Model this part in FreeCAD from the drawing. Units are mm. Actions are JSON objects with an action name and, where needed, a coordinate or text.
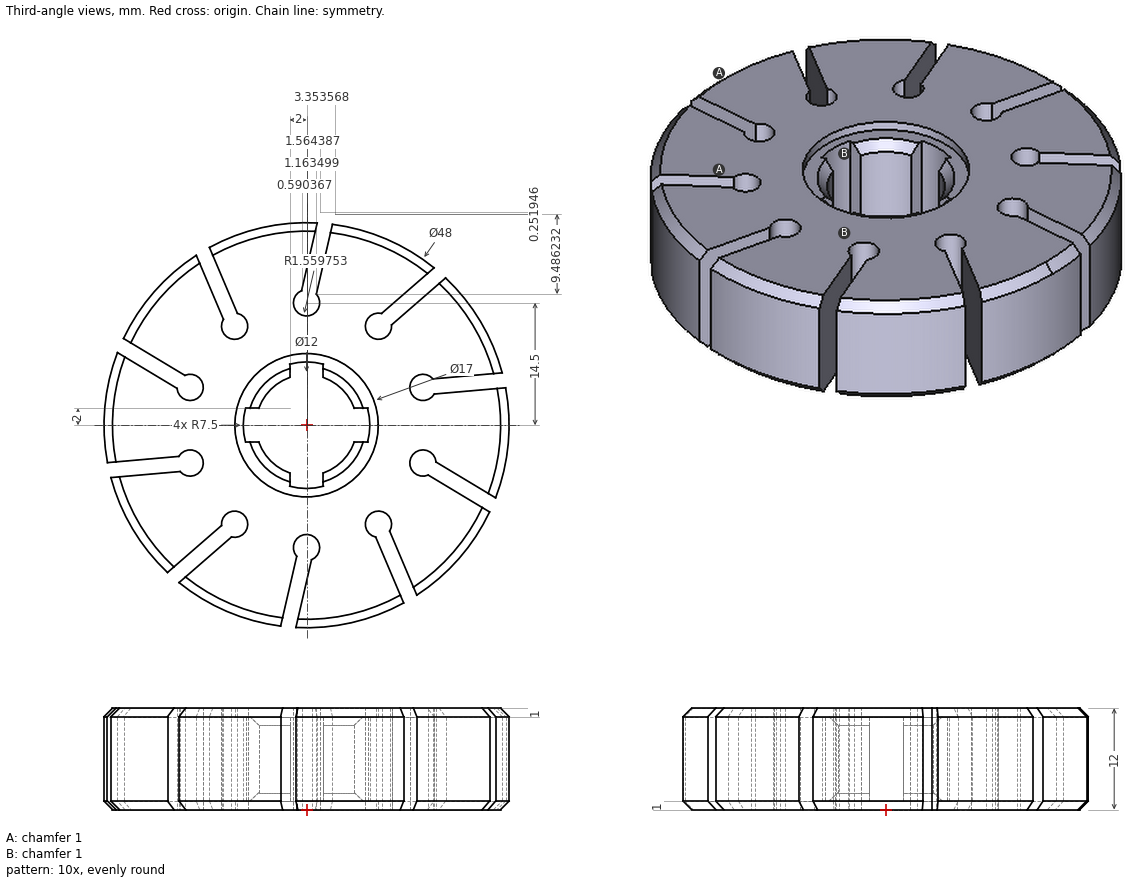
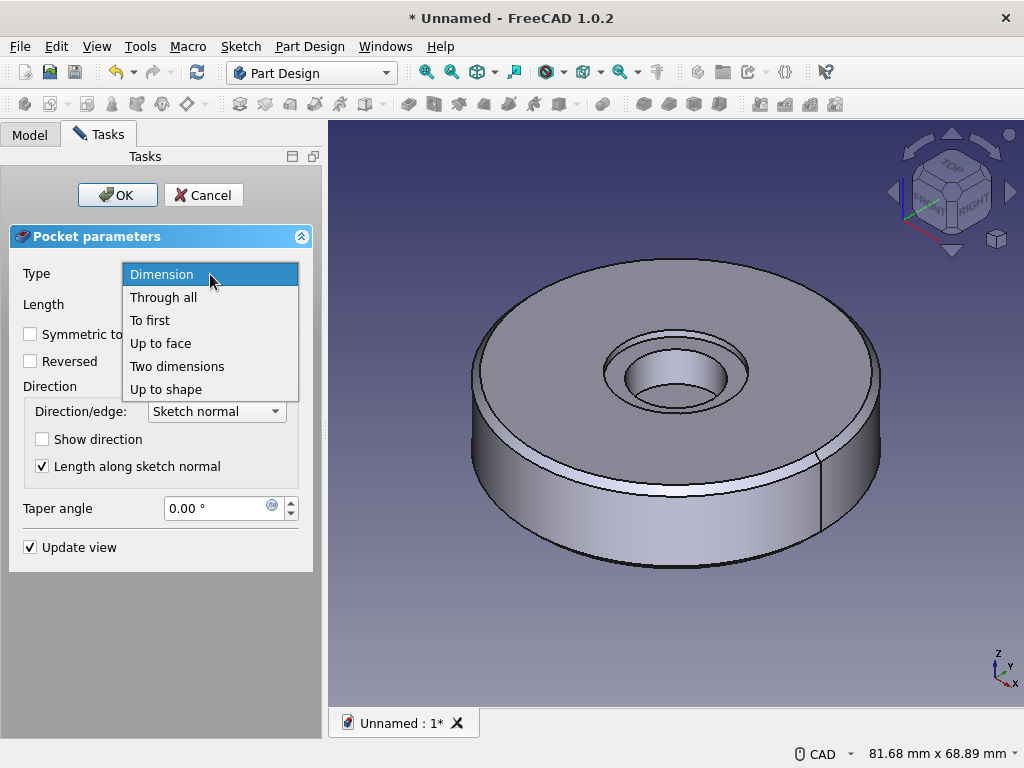
{"action": "left_click", "coordinate": [208, 298]}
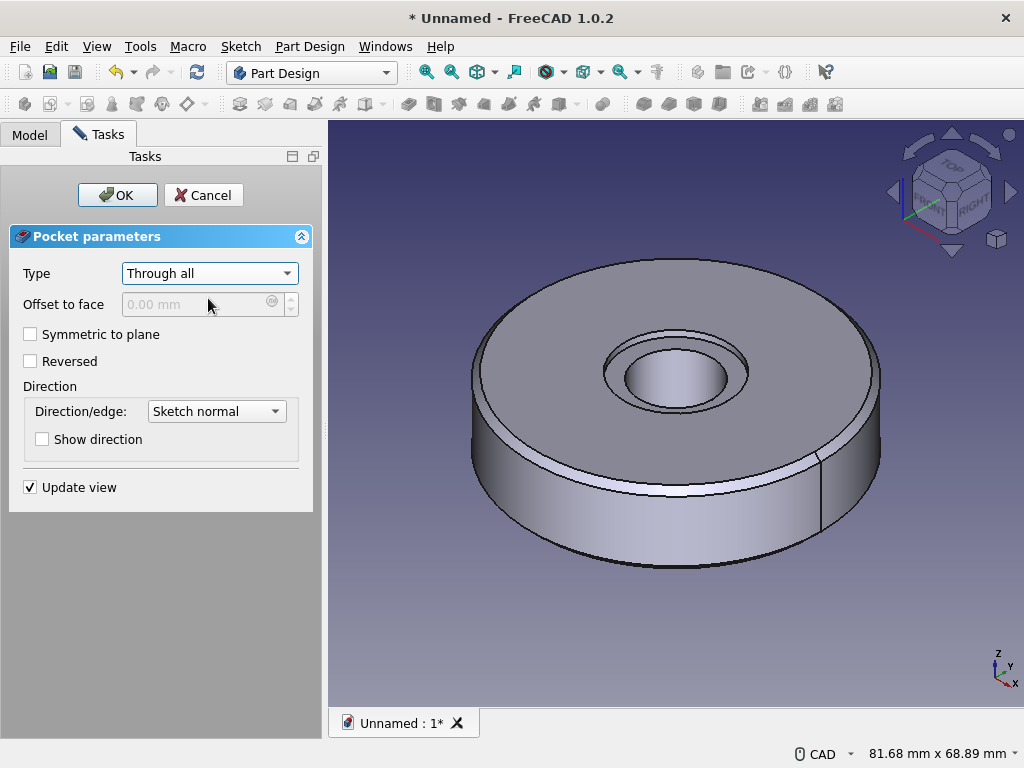
{"action": "left_click", "coordinate": [118, 195]}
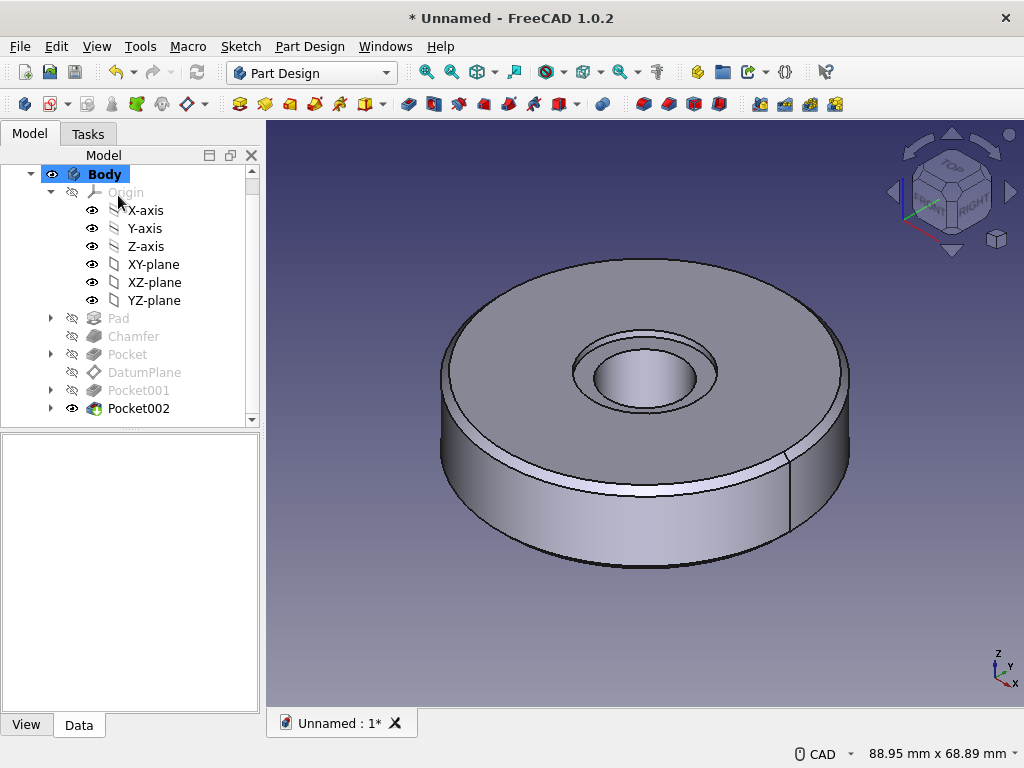
{"action": "left_click", "coordinate": [609, 357]}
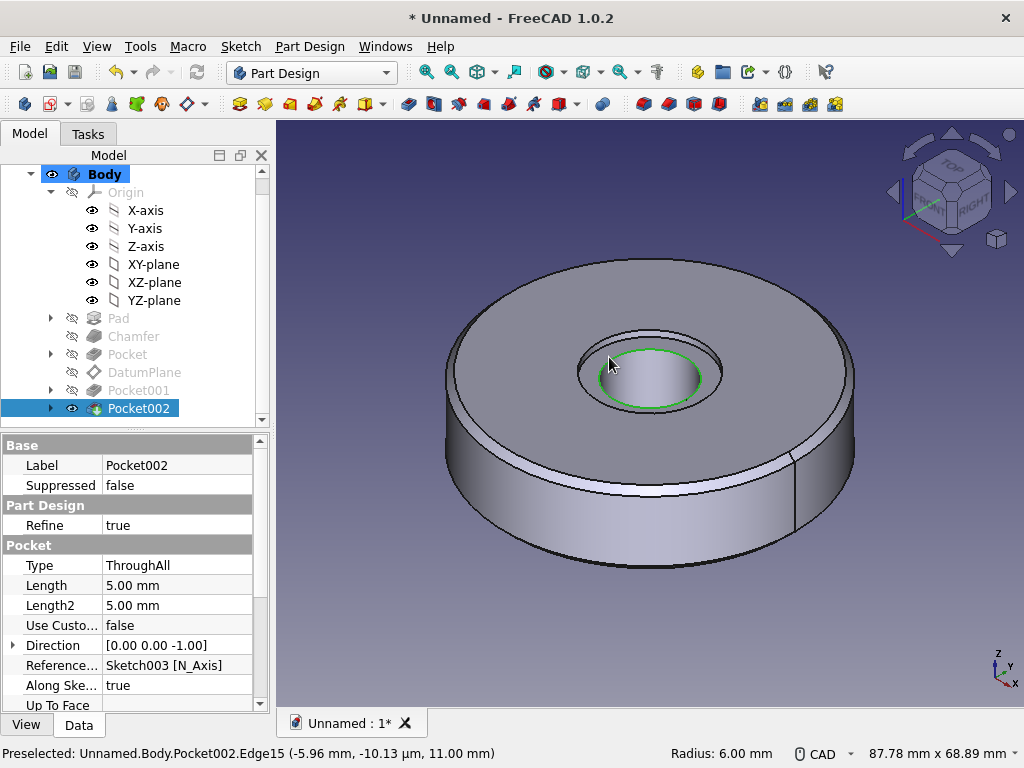
{"action": "key", "text": "2"}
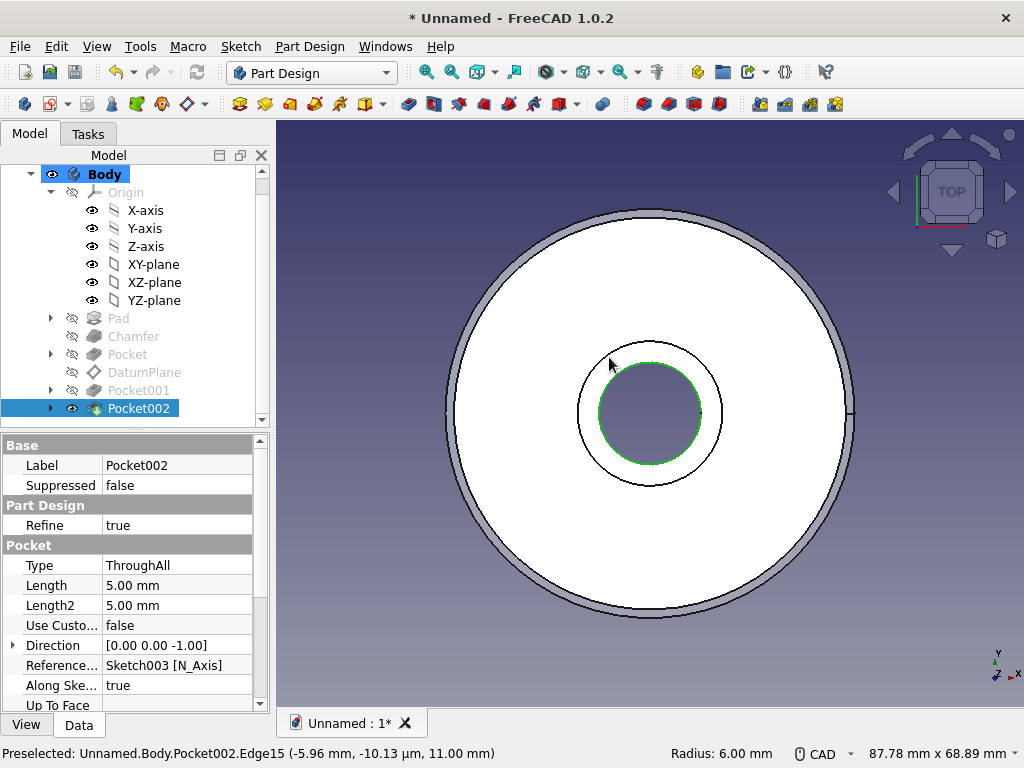
{"action": "key", "text": "0"}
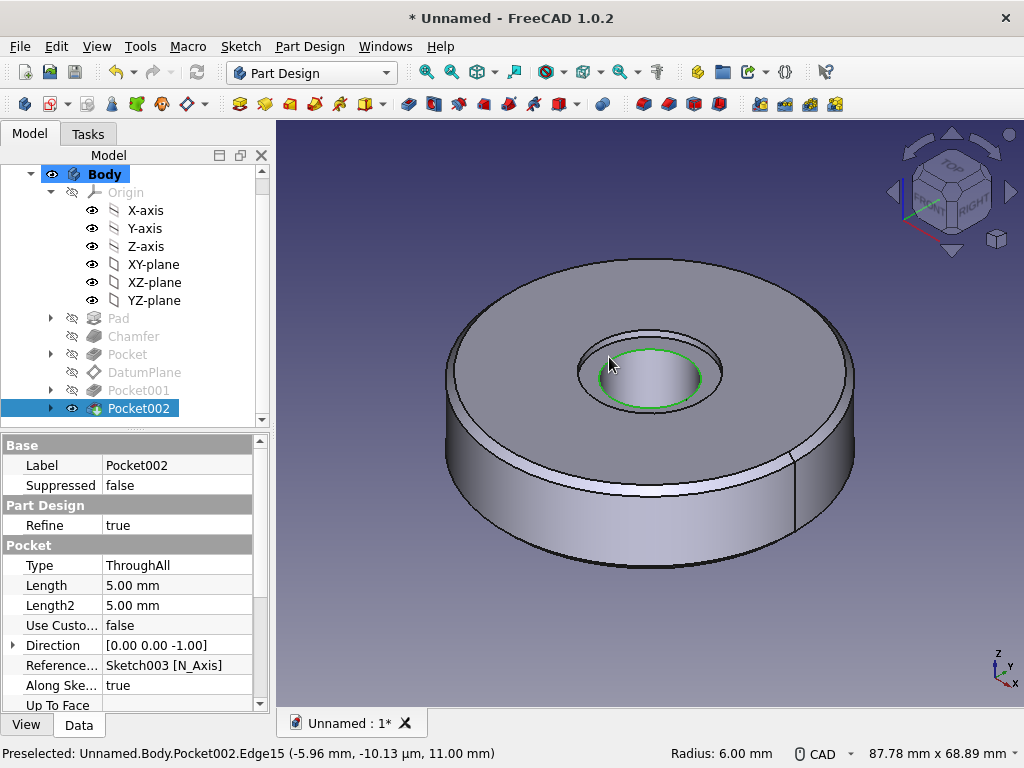
{"action": "key", "text": "1"}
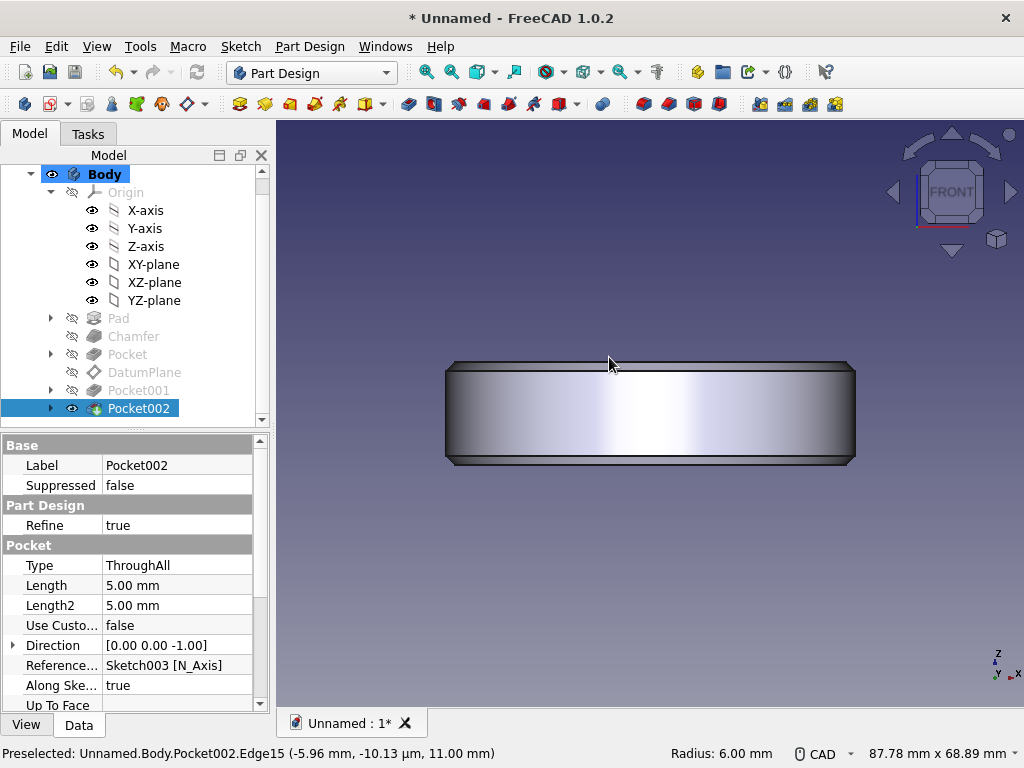
{"action": "key", "text": "3"}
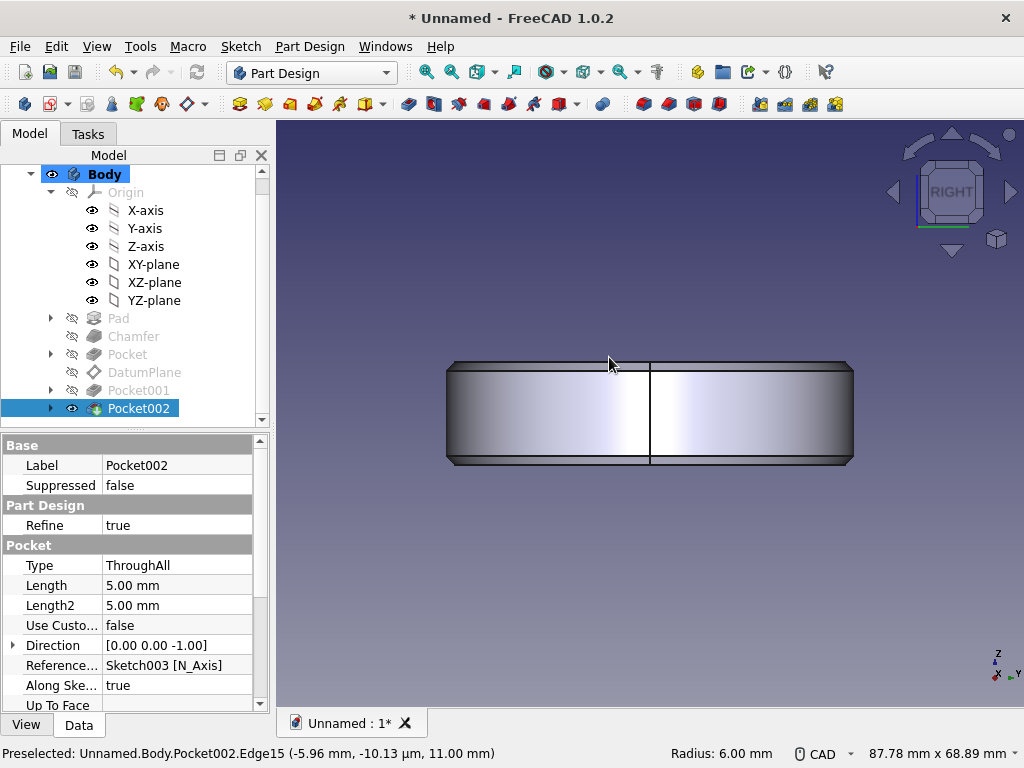
{"action": "key", "text": "5"}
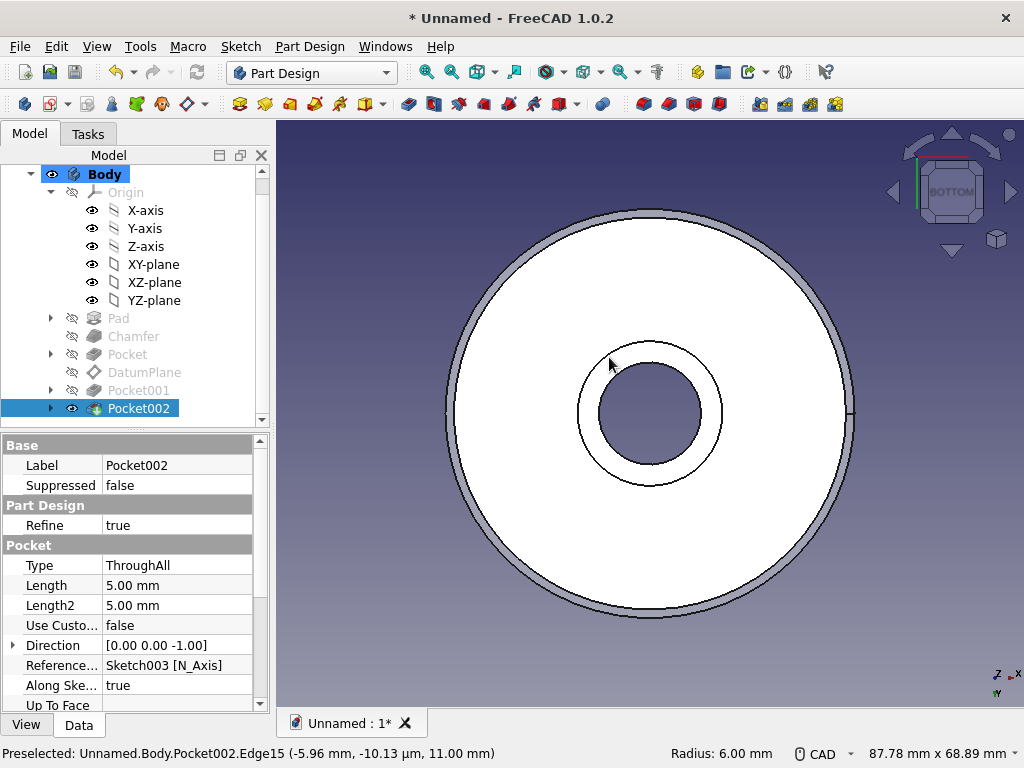
{"action": "left_click", "coordinate": [599, 413], "text": "ctrl"}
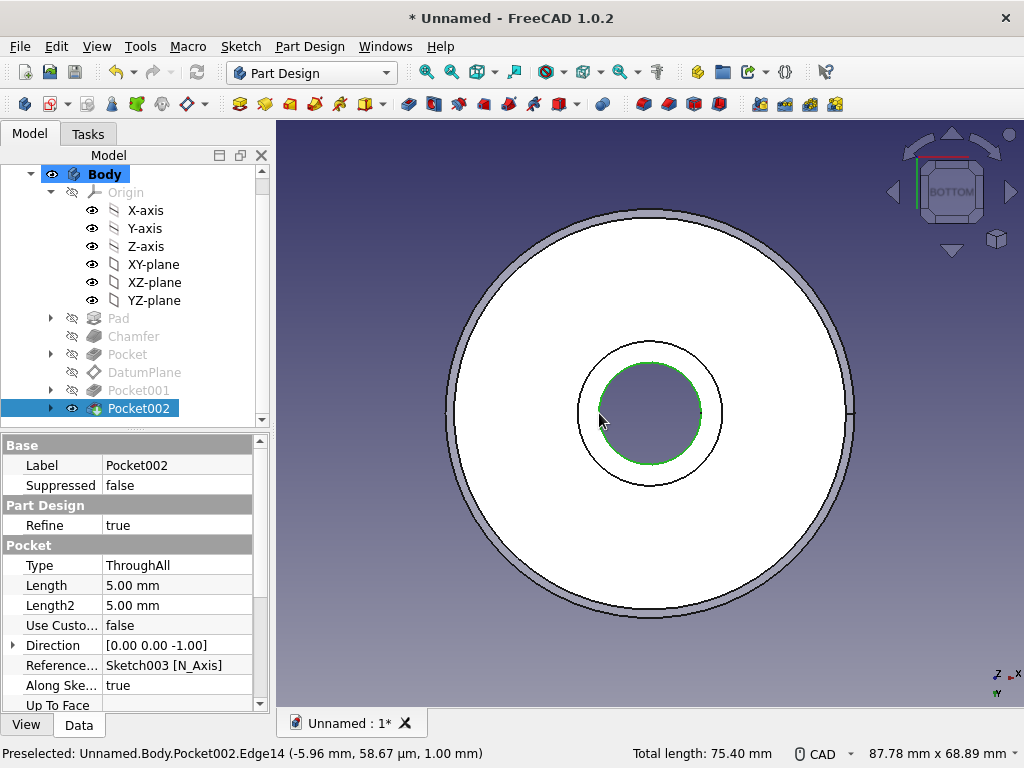
{"action": "left_click", "coordinate": [669, 104]}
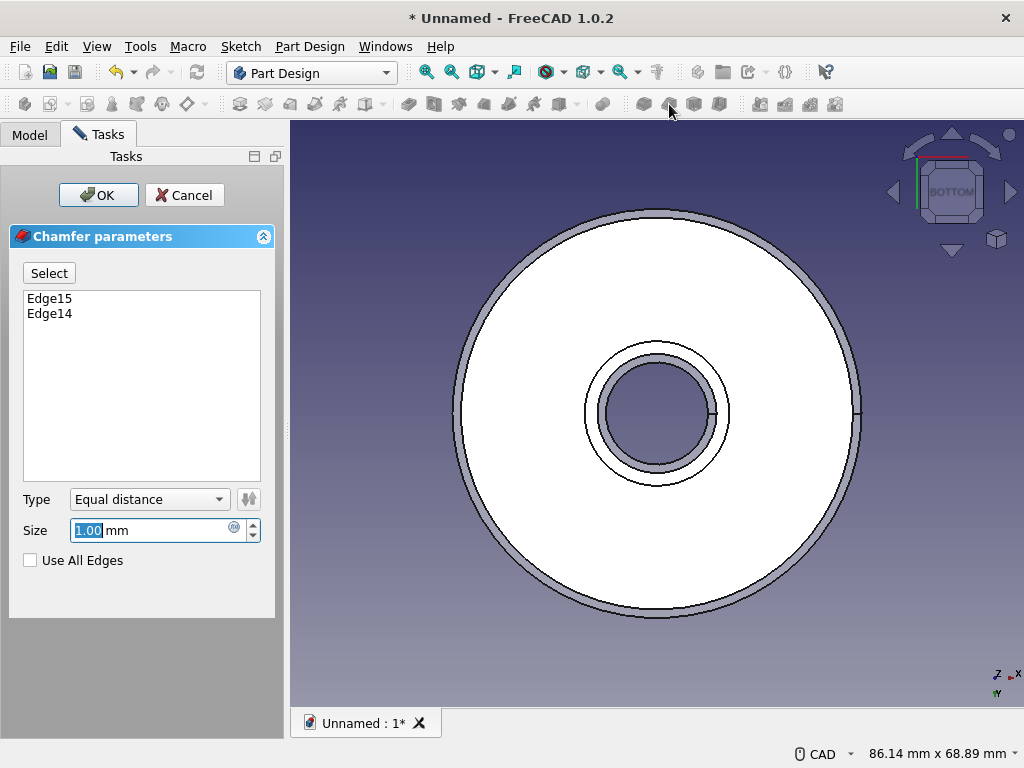
{"action": "type", "text": "1"}
{"action": "key", "text": "Tab"}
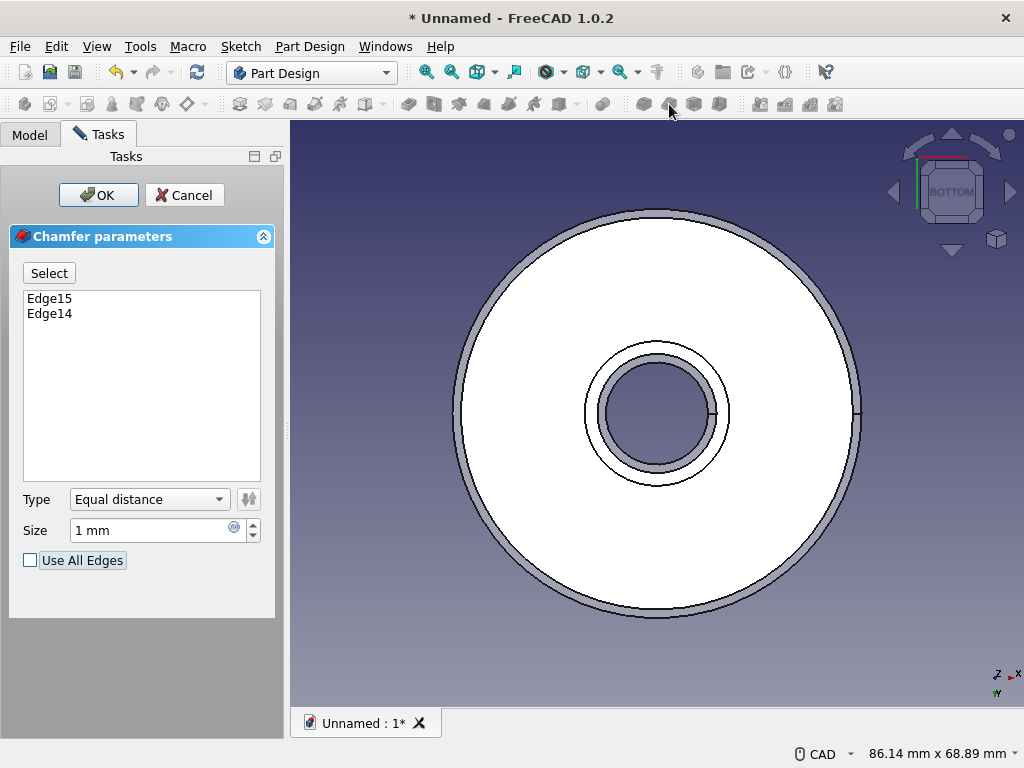
{"action": "left_click", "coordinate": [99, 195]}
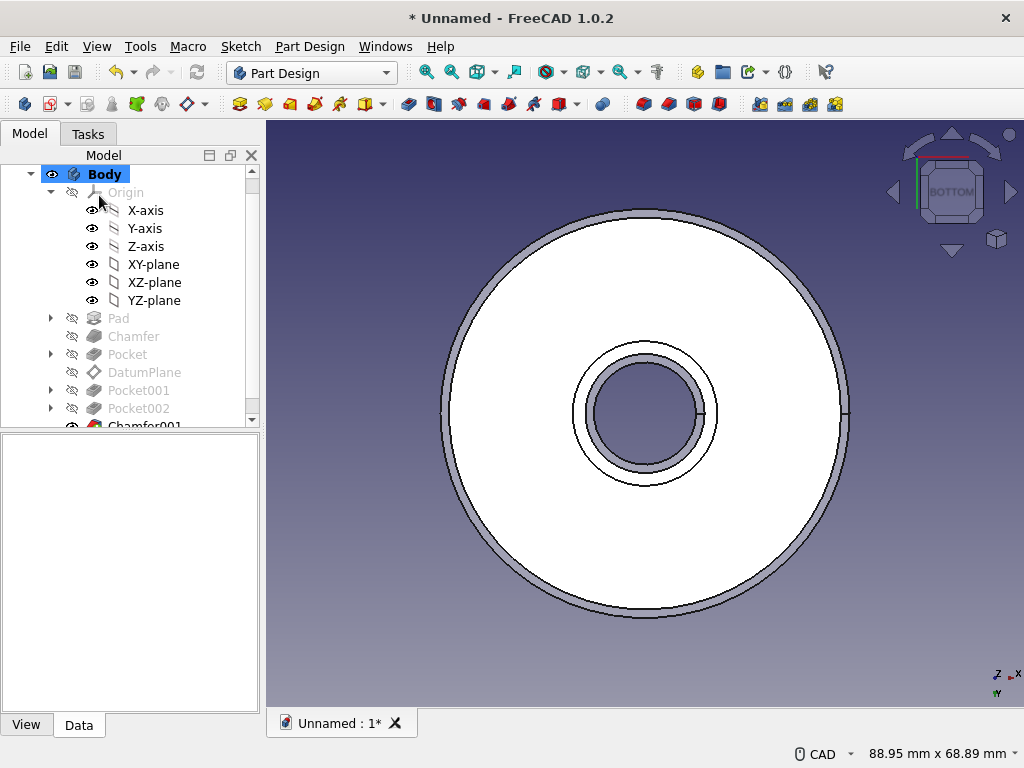
{"action": "key", "text": "0"}